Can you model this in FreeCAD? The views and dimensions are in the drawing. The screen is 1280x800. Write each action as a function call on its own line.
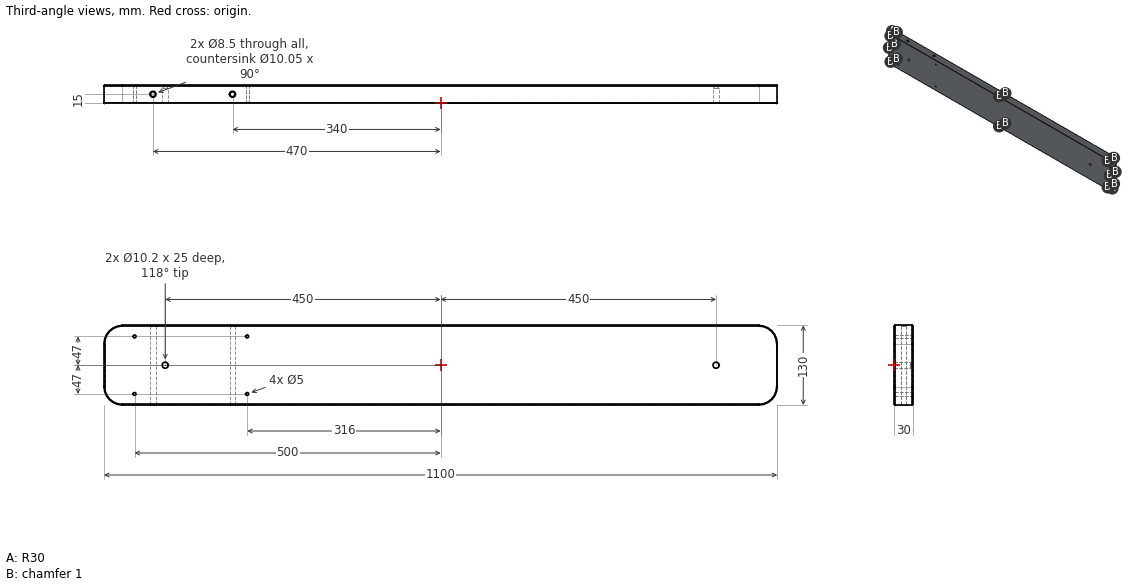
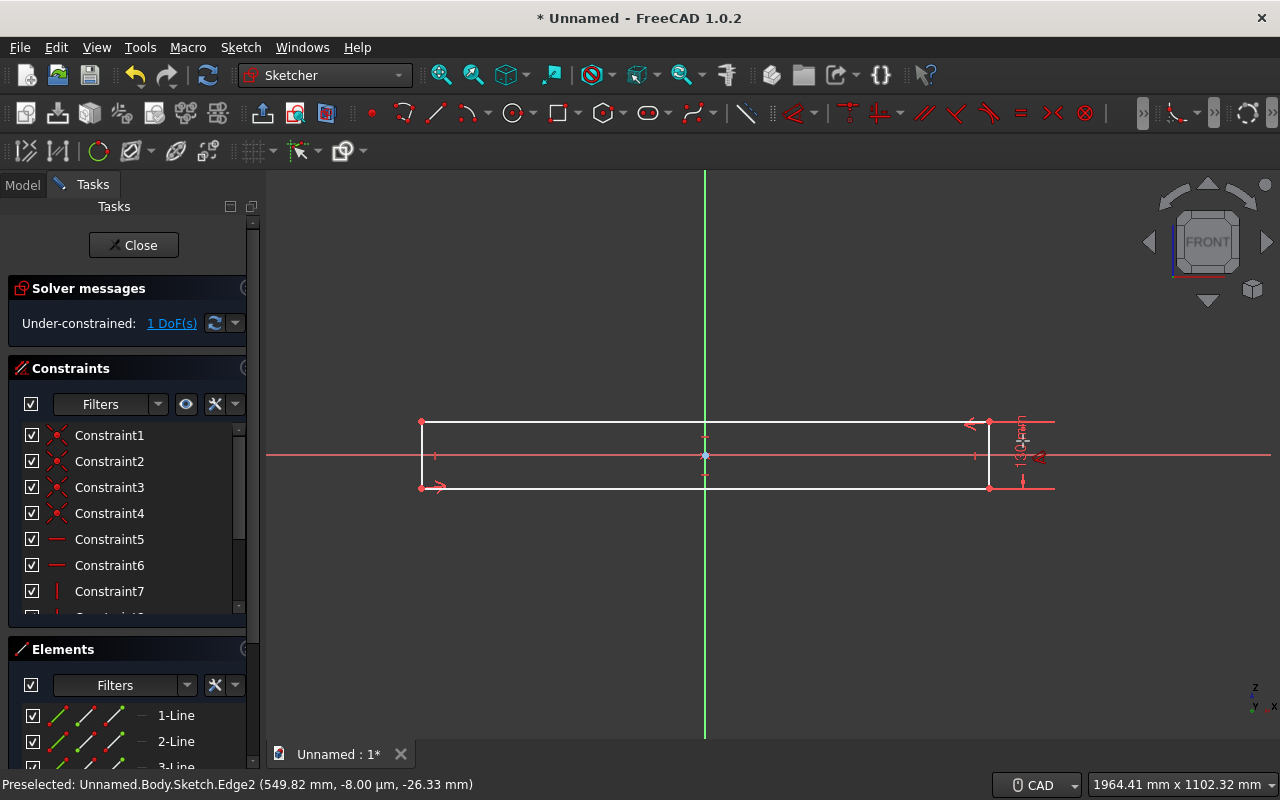
click(592, 489)
click(575, 523)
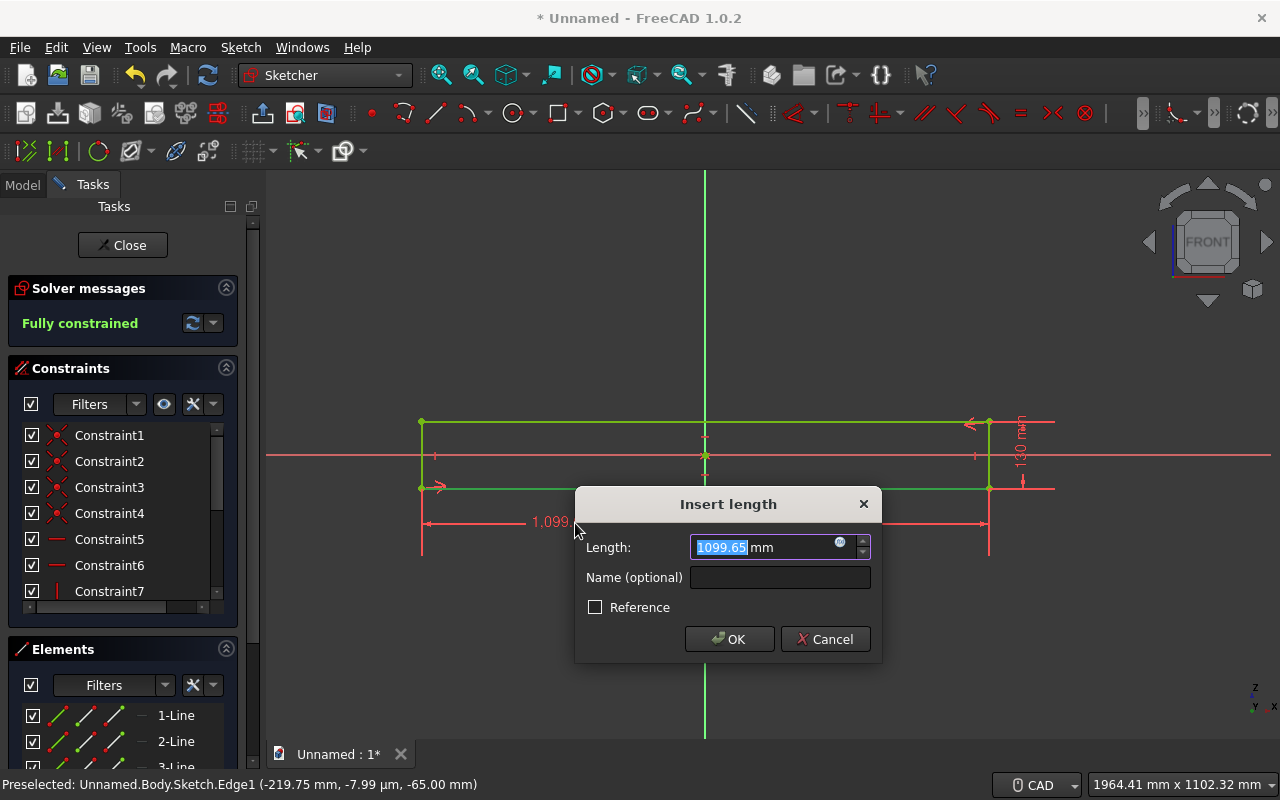
text(1100)
key(Return)
key(Escape)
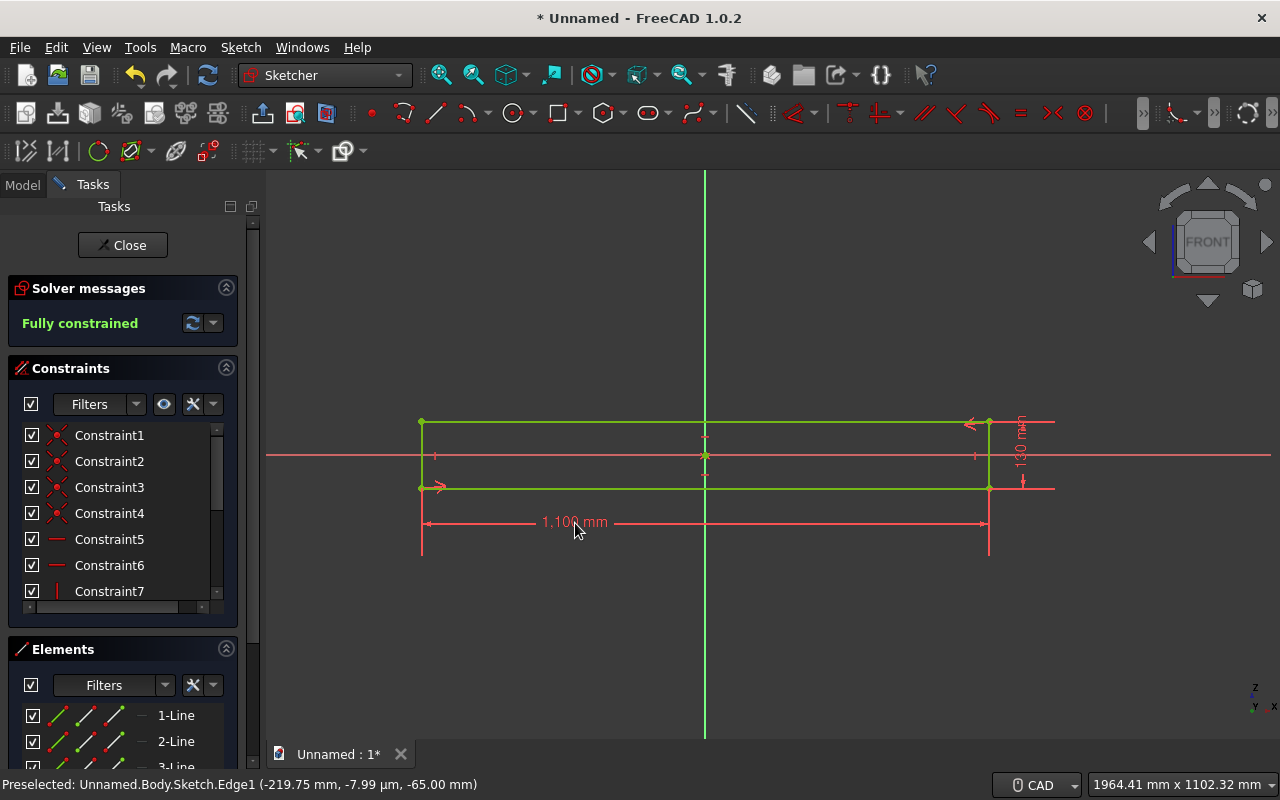
click(123, 245)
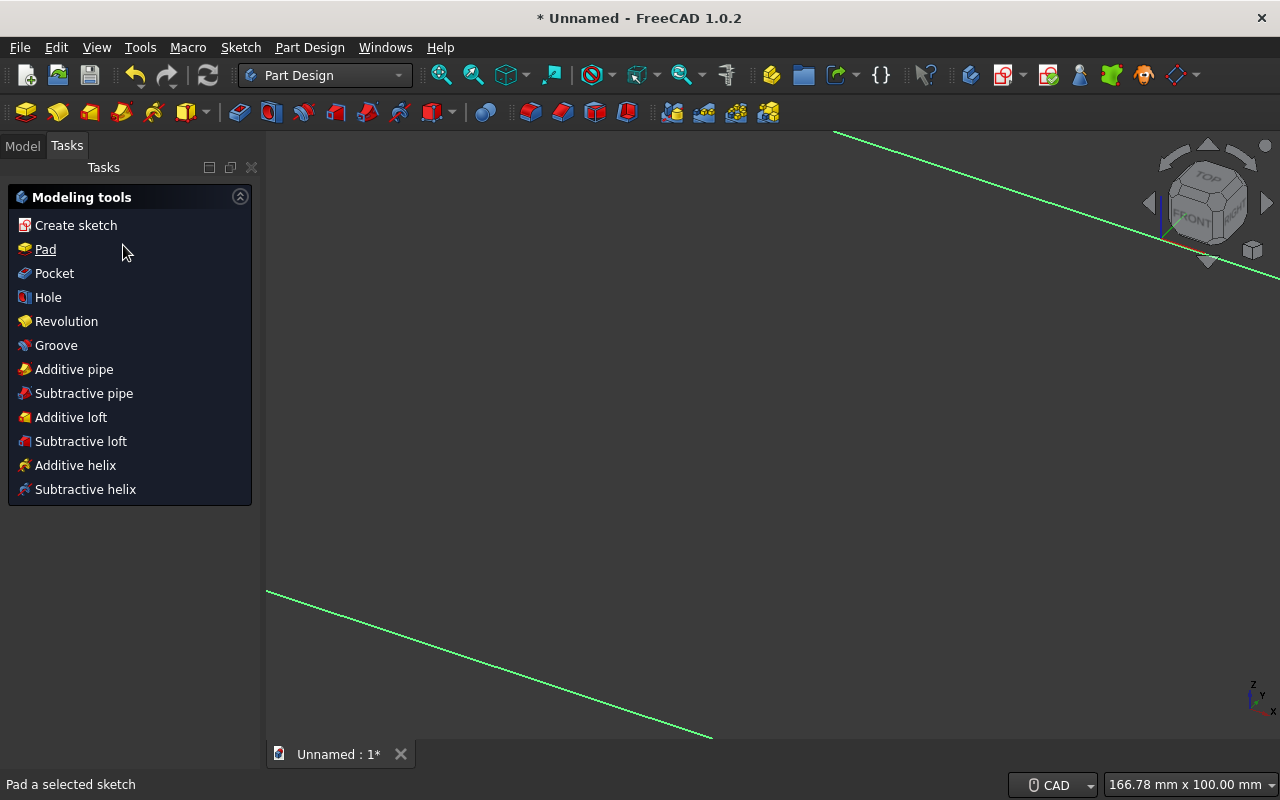
click(26, 112)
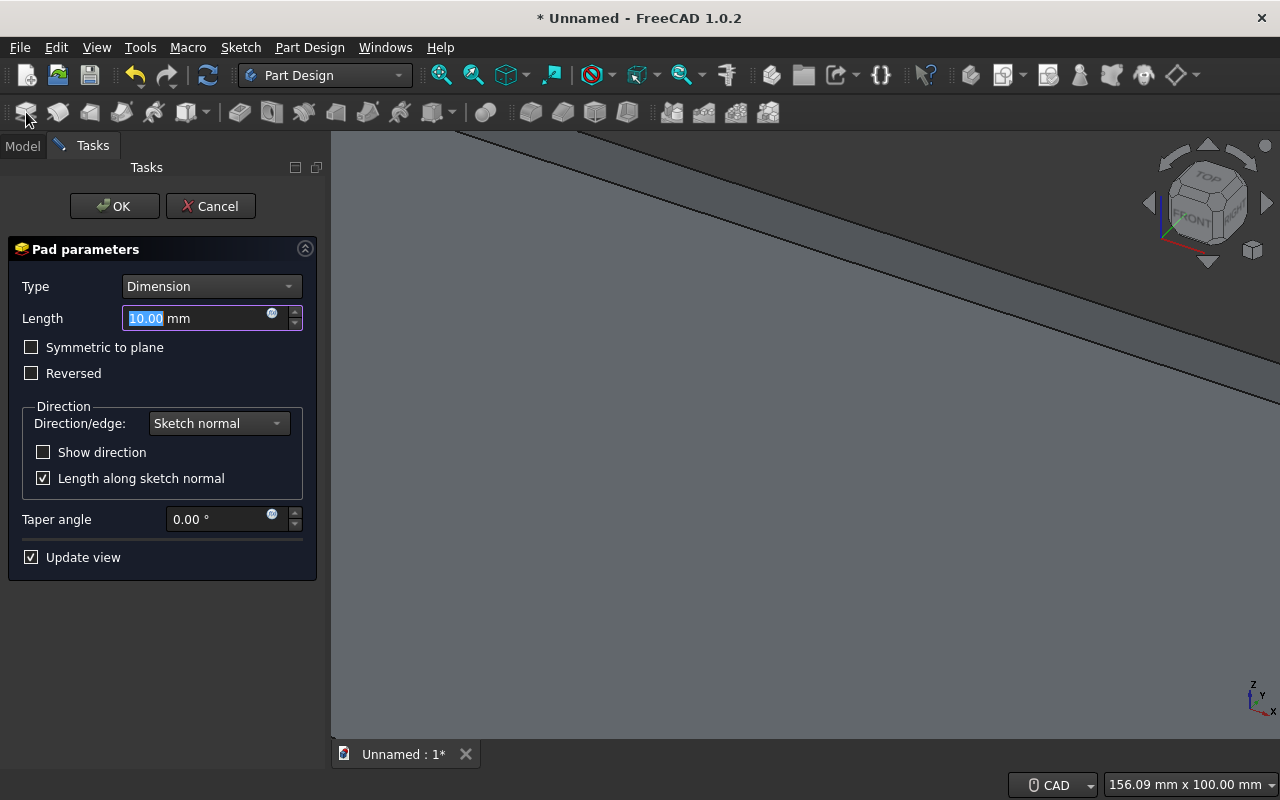
text(30)
key(Tab)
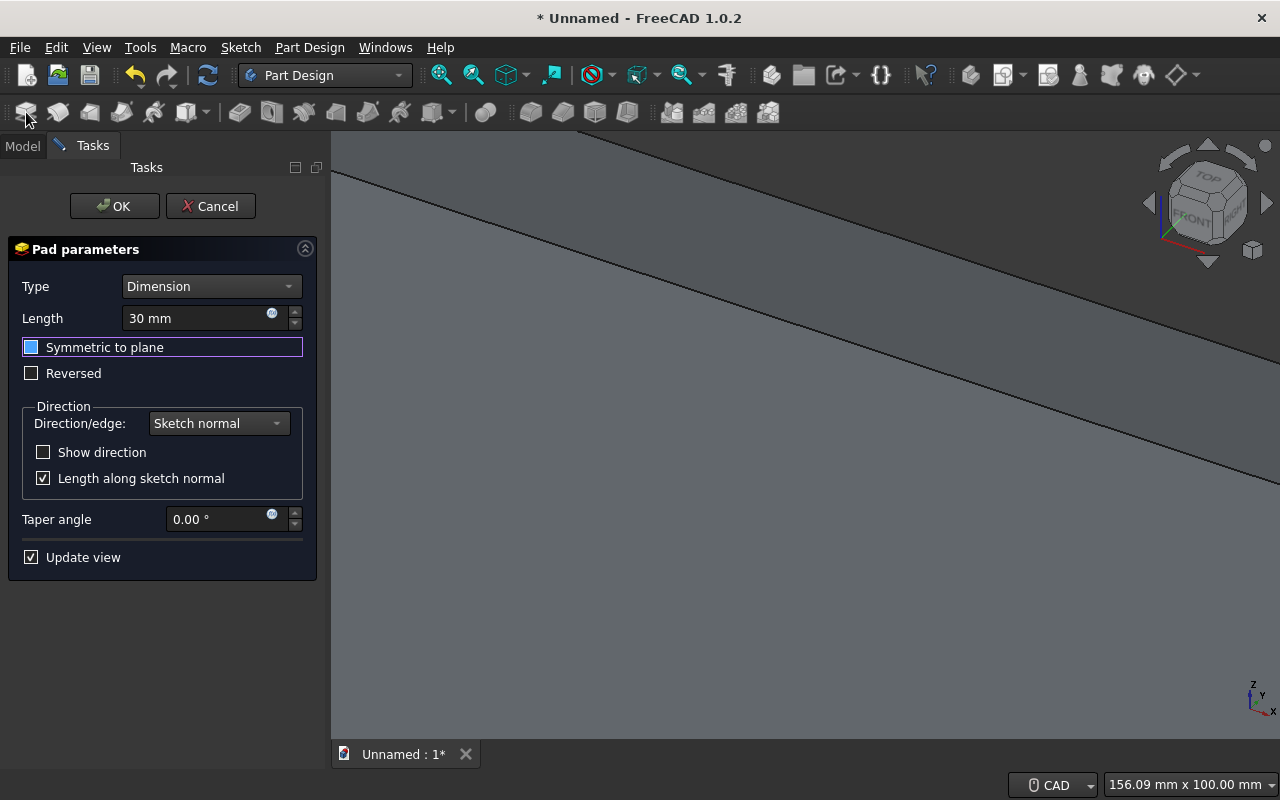
click(30, 373)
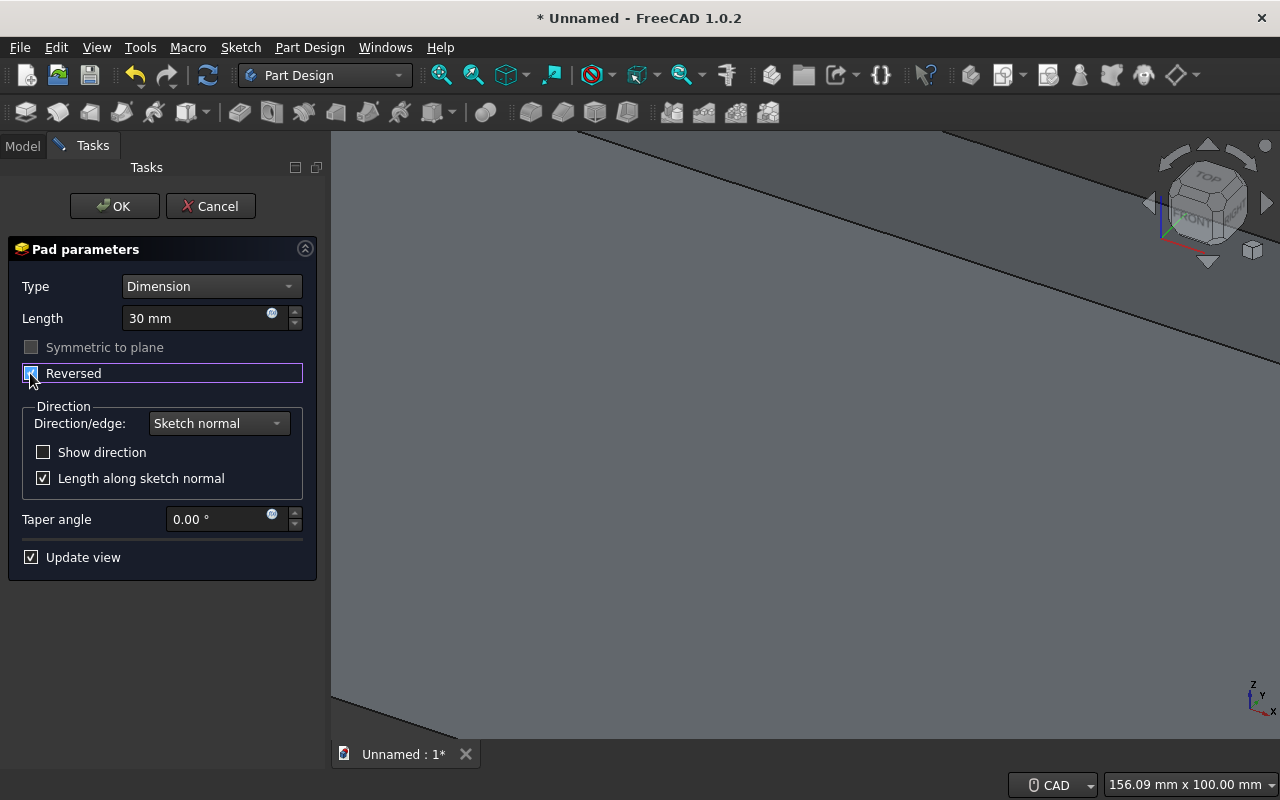
click(115, 206)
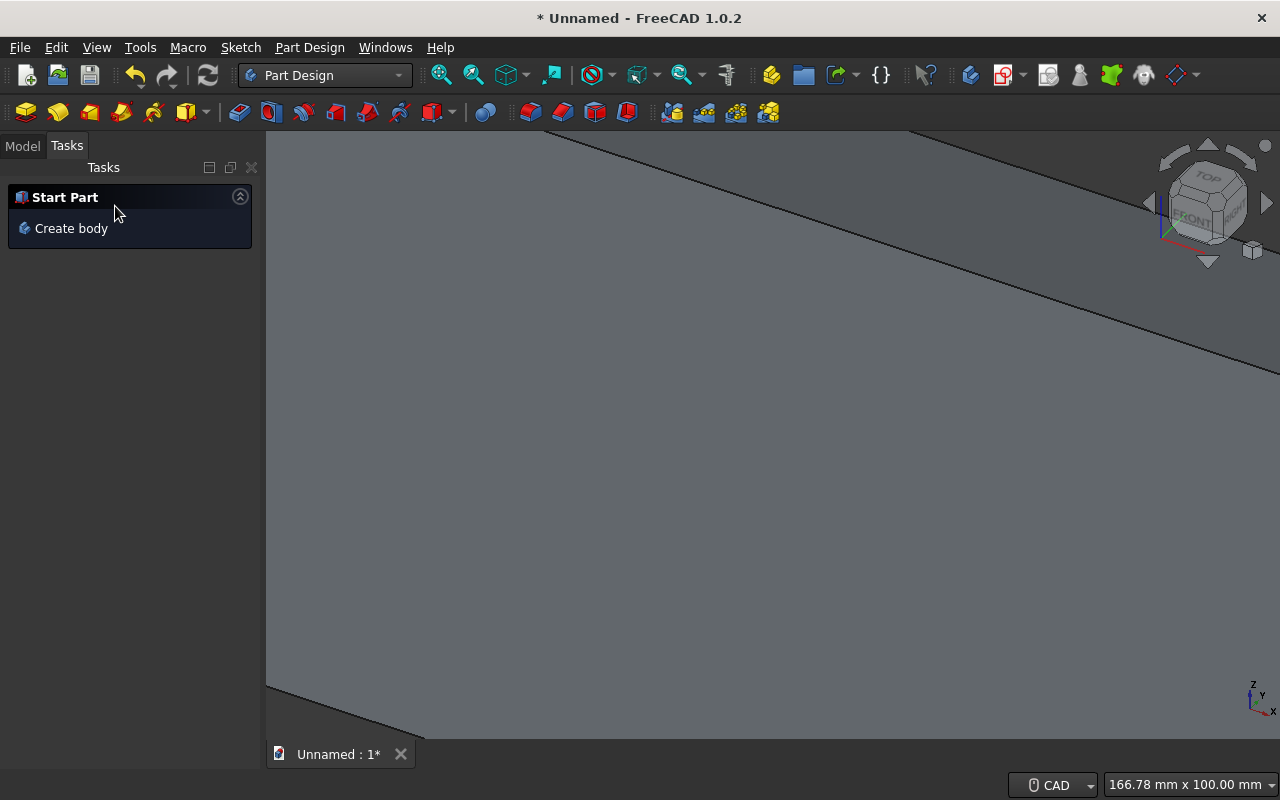
click(442, 76)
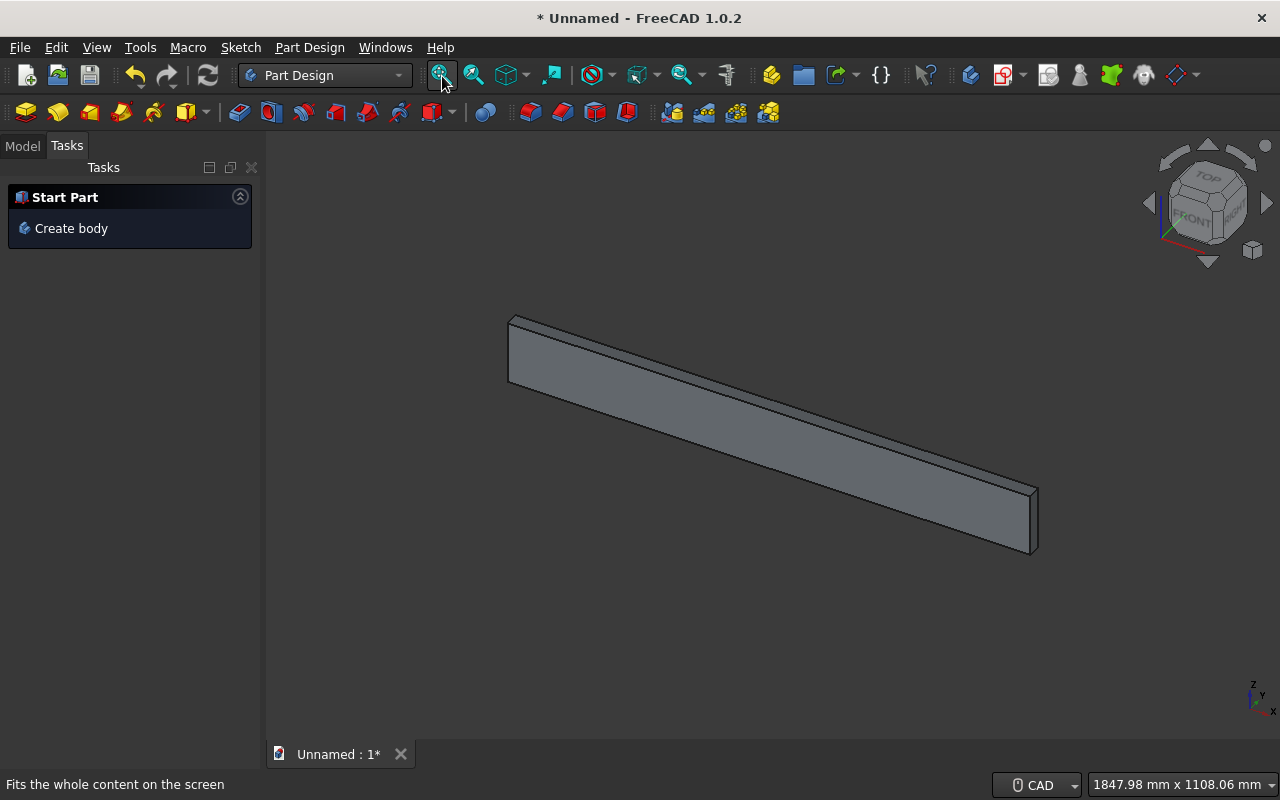
key(4)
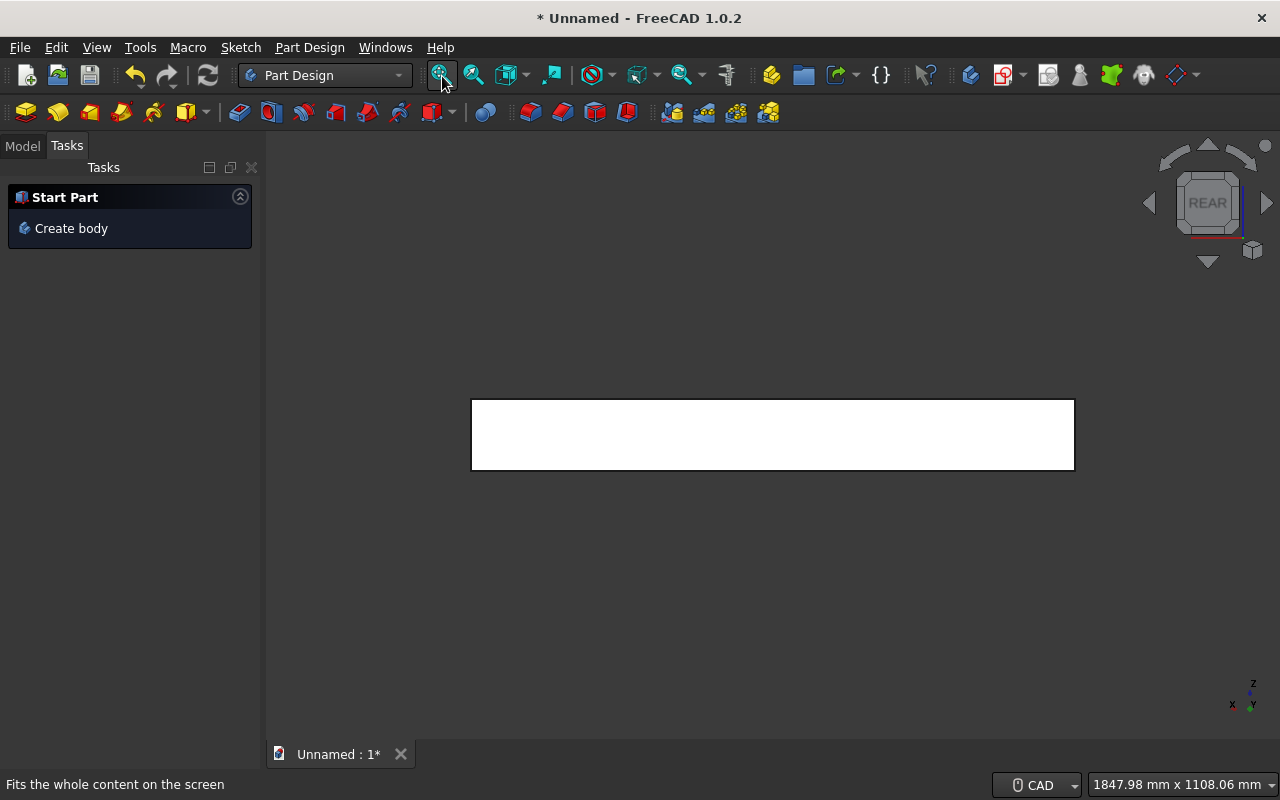
click(514, 434)